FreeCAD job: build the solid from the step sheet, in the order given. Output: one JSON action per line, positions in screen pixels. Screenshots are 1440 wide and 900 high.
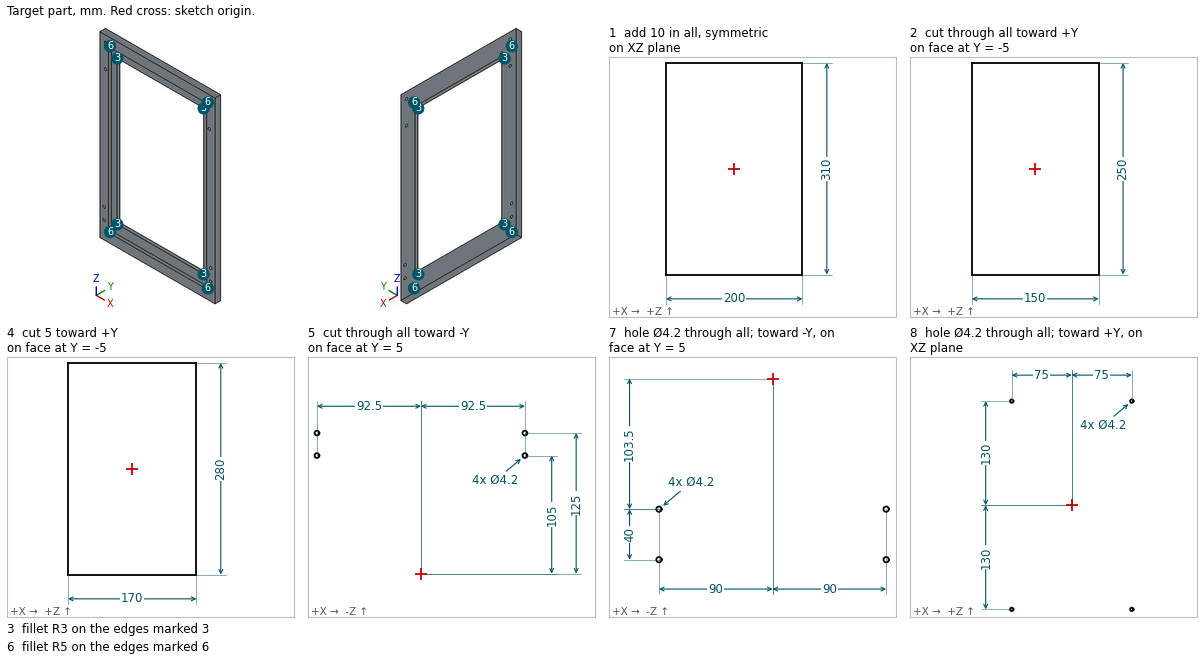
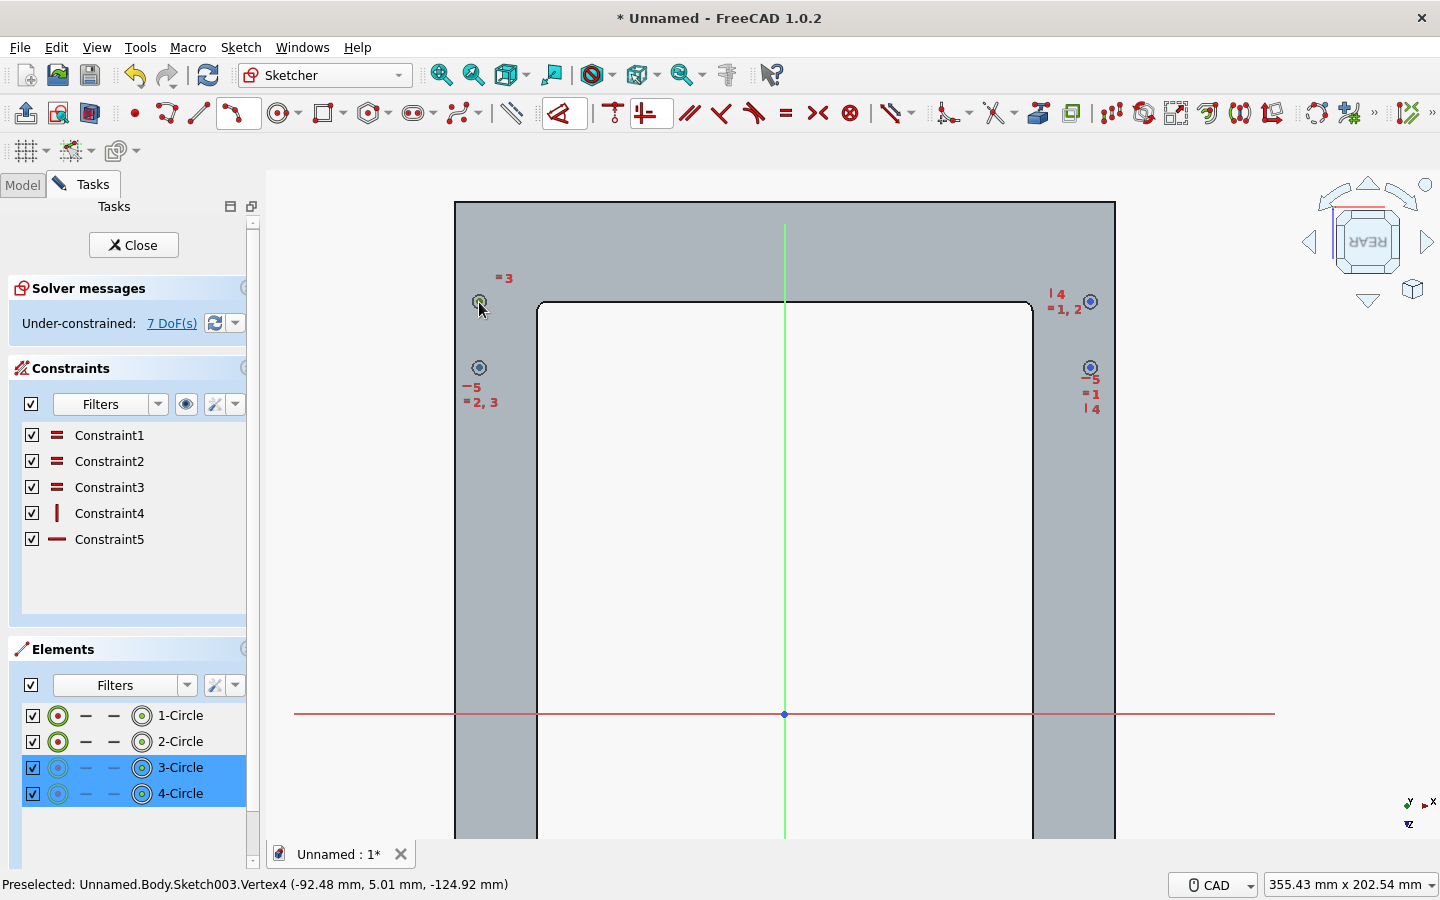
{"action": "key", "text": "v"}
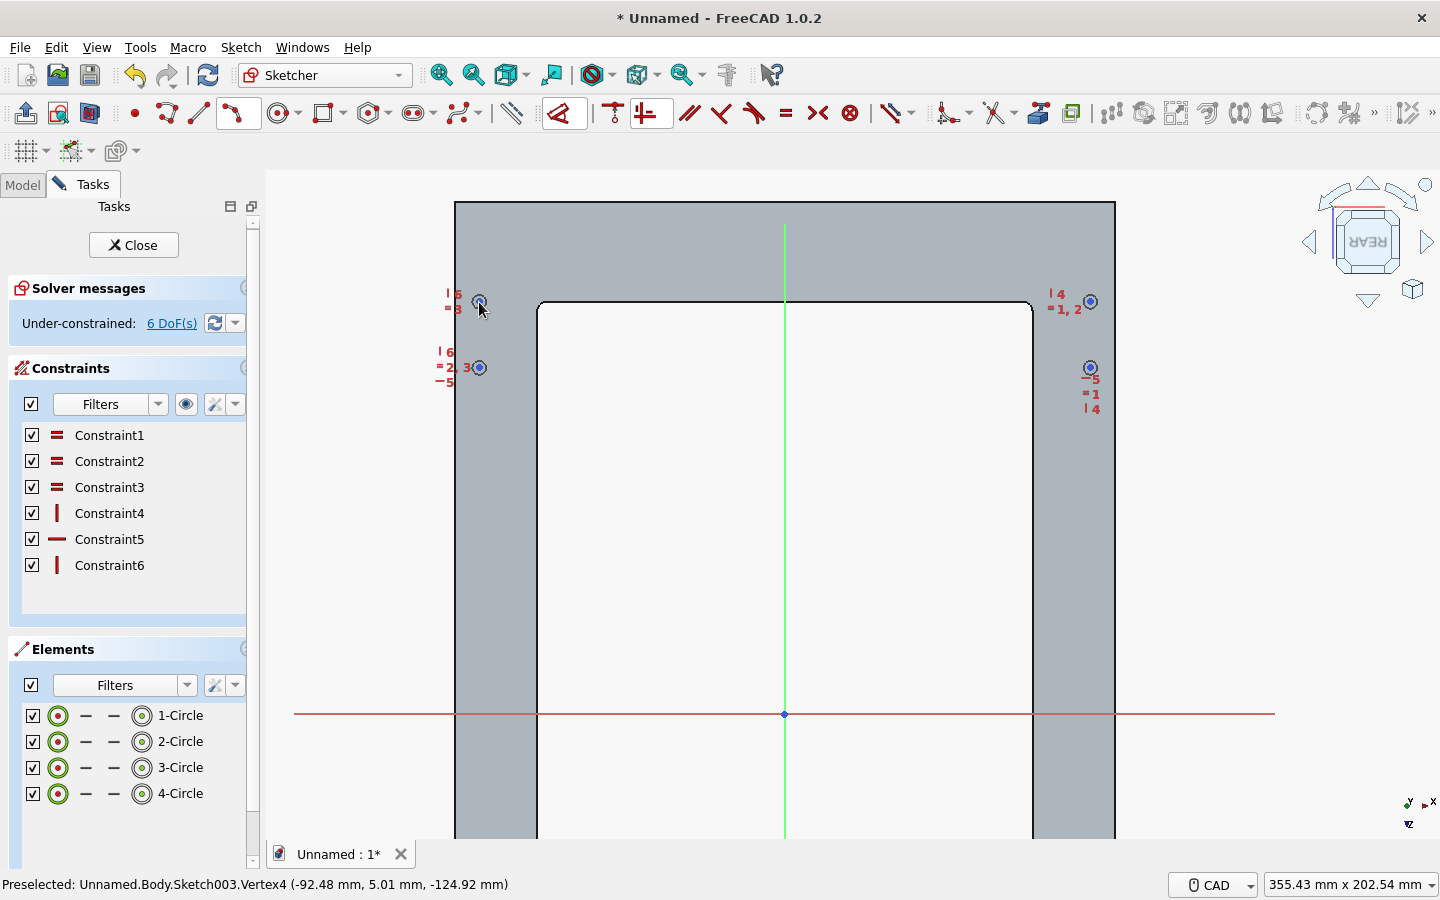
{"action": "left_click", "coordinate": [1090, 302]}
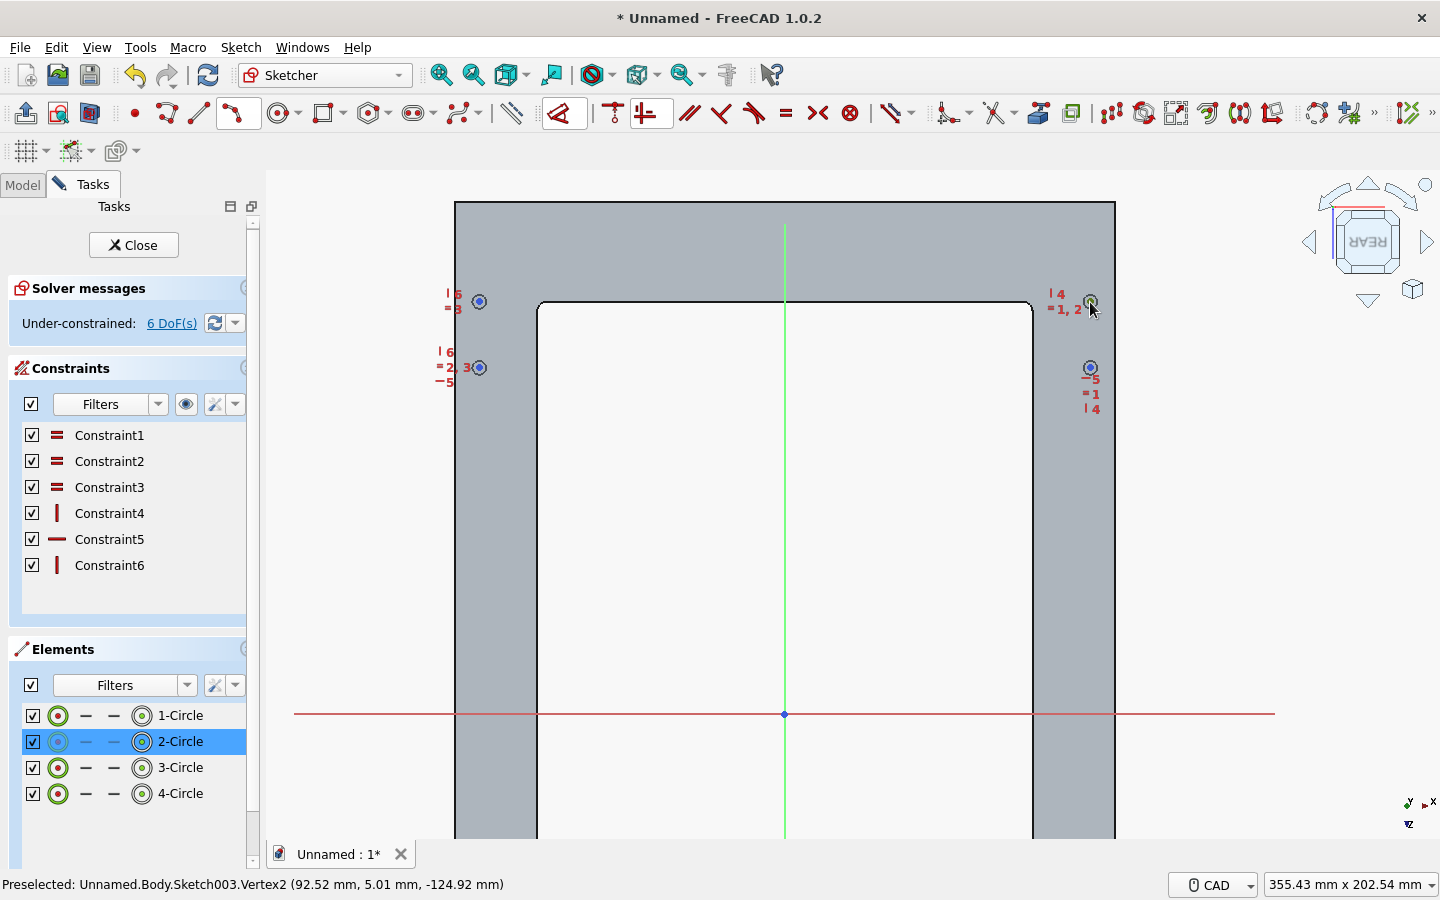
{"action": "left_click", "coordinate": [479, 302]}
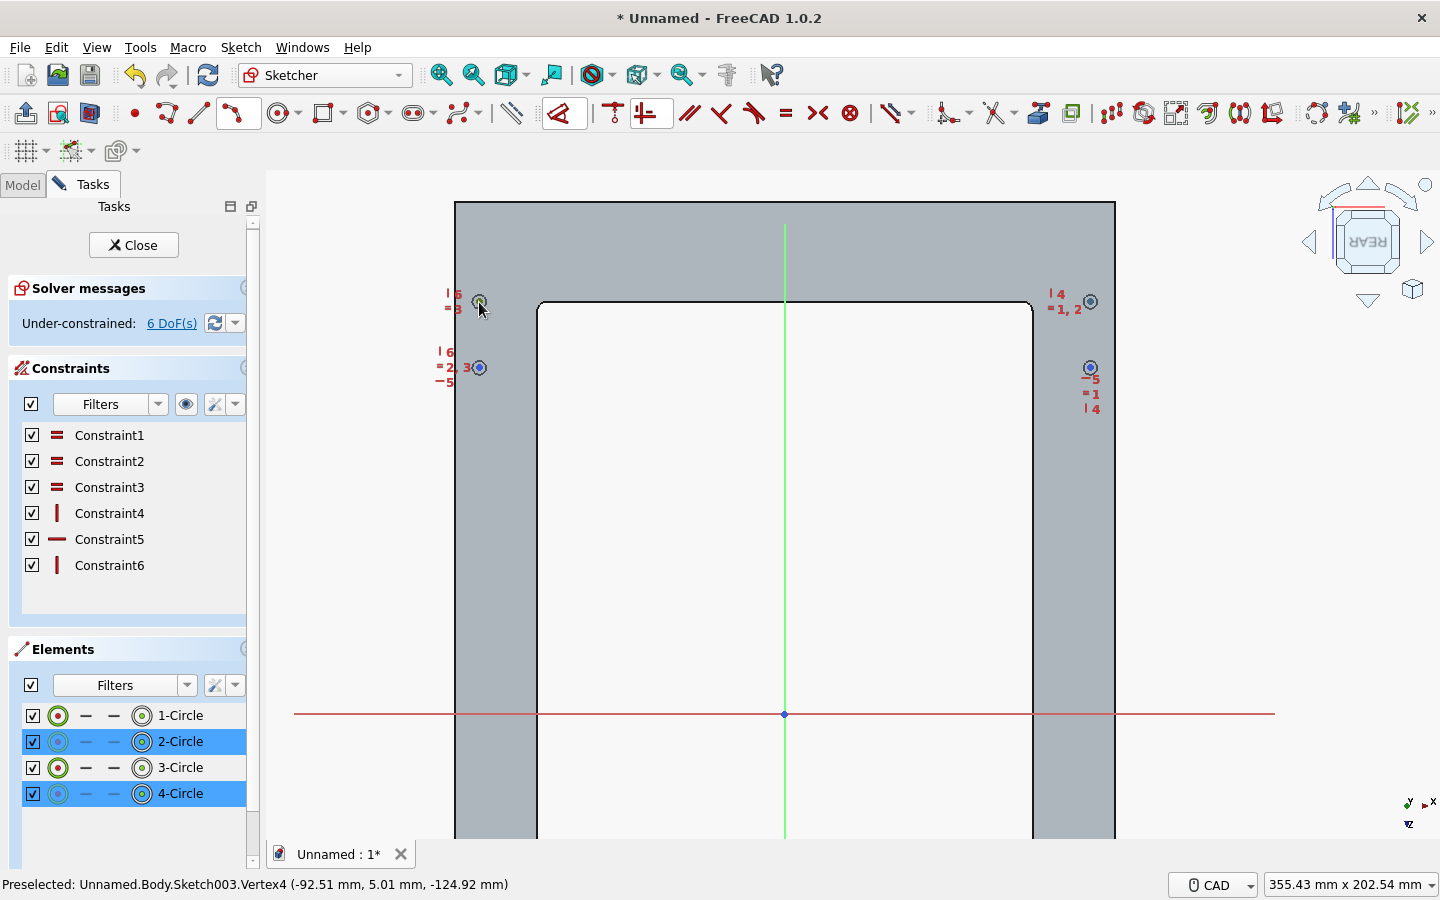
{"action": "key", "text": "h"}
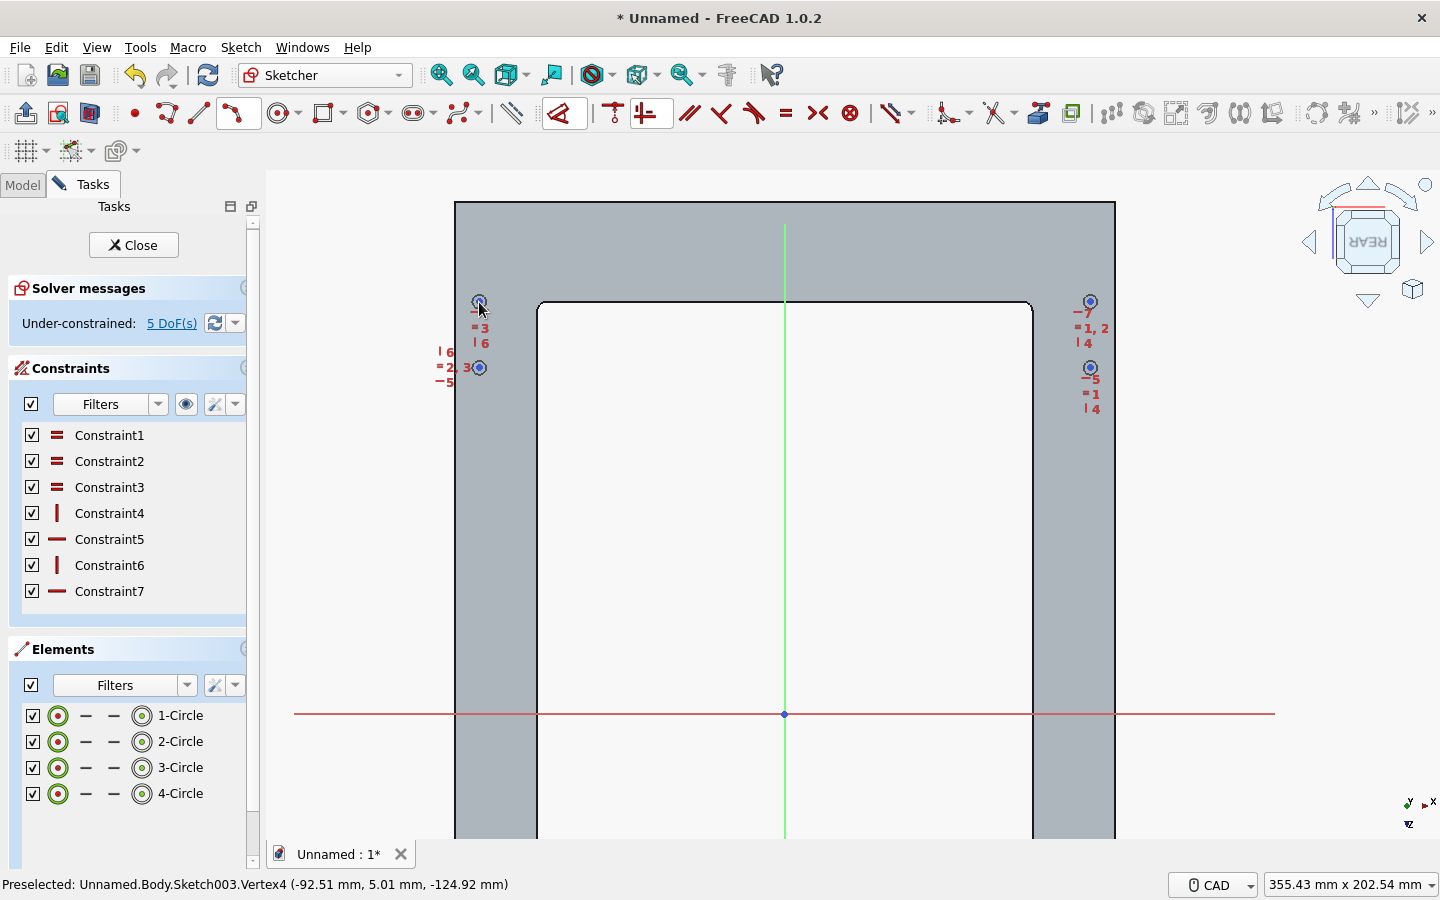
{"action": "scroll", "coordinate": [1091, 361], "scroll_direction": "up", "scroll_amount": 6}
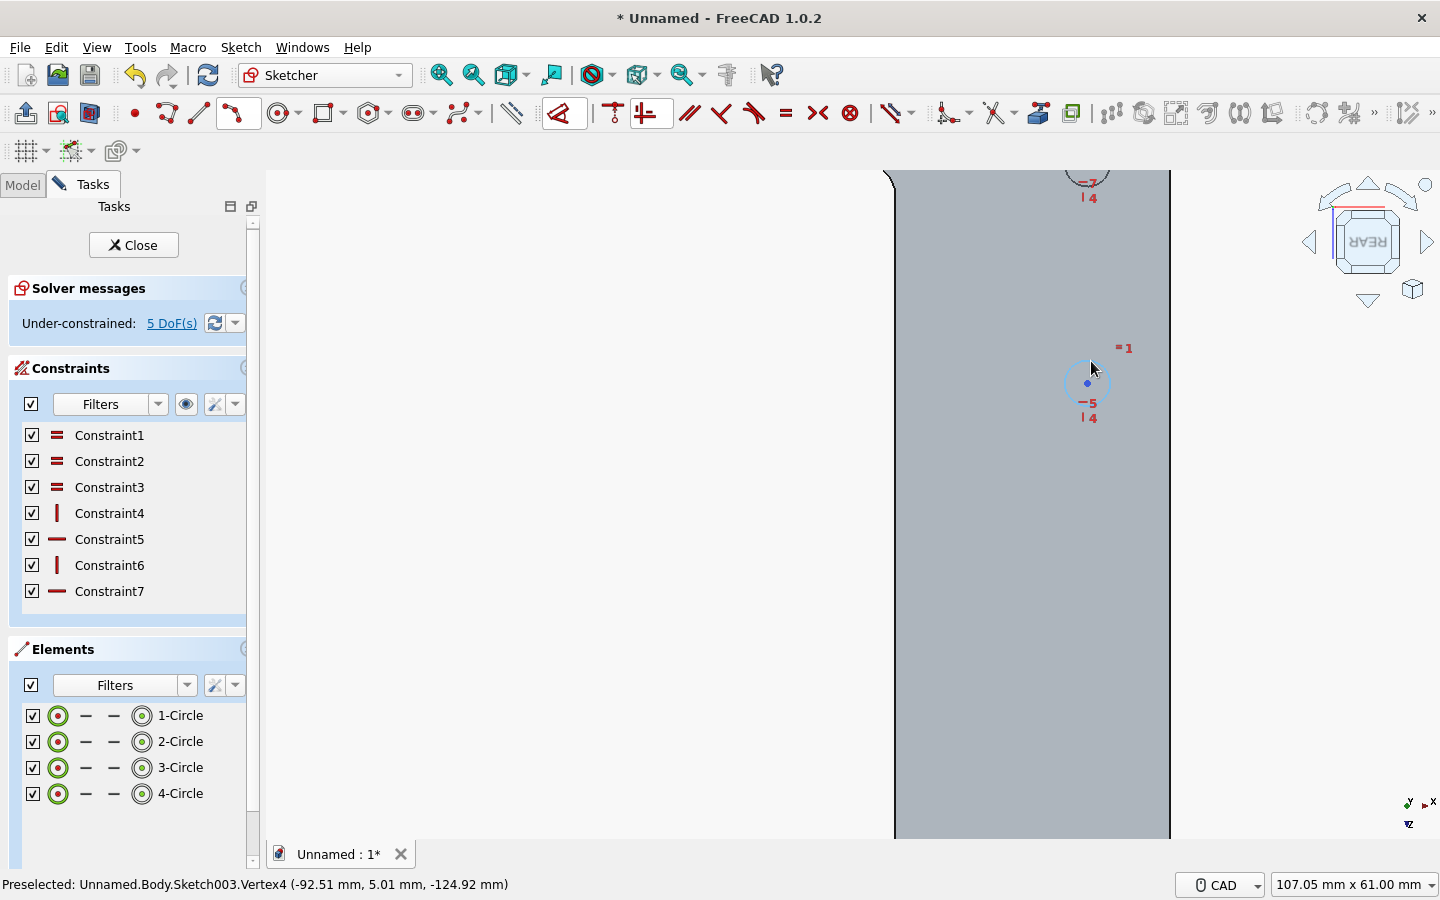
{"action": "left_click", "coordinate": [1088, 361]}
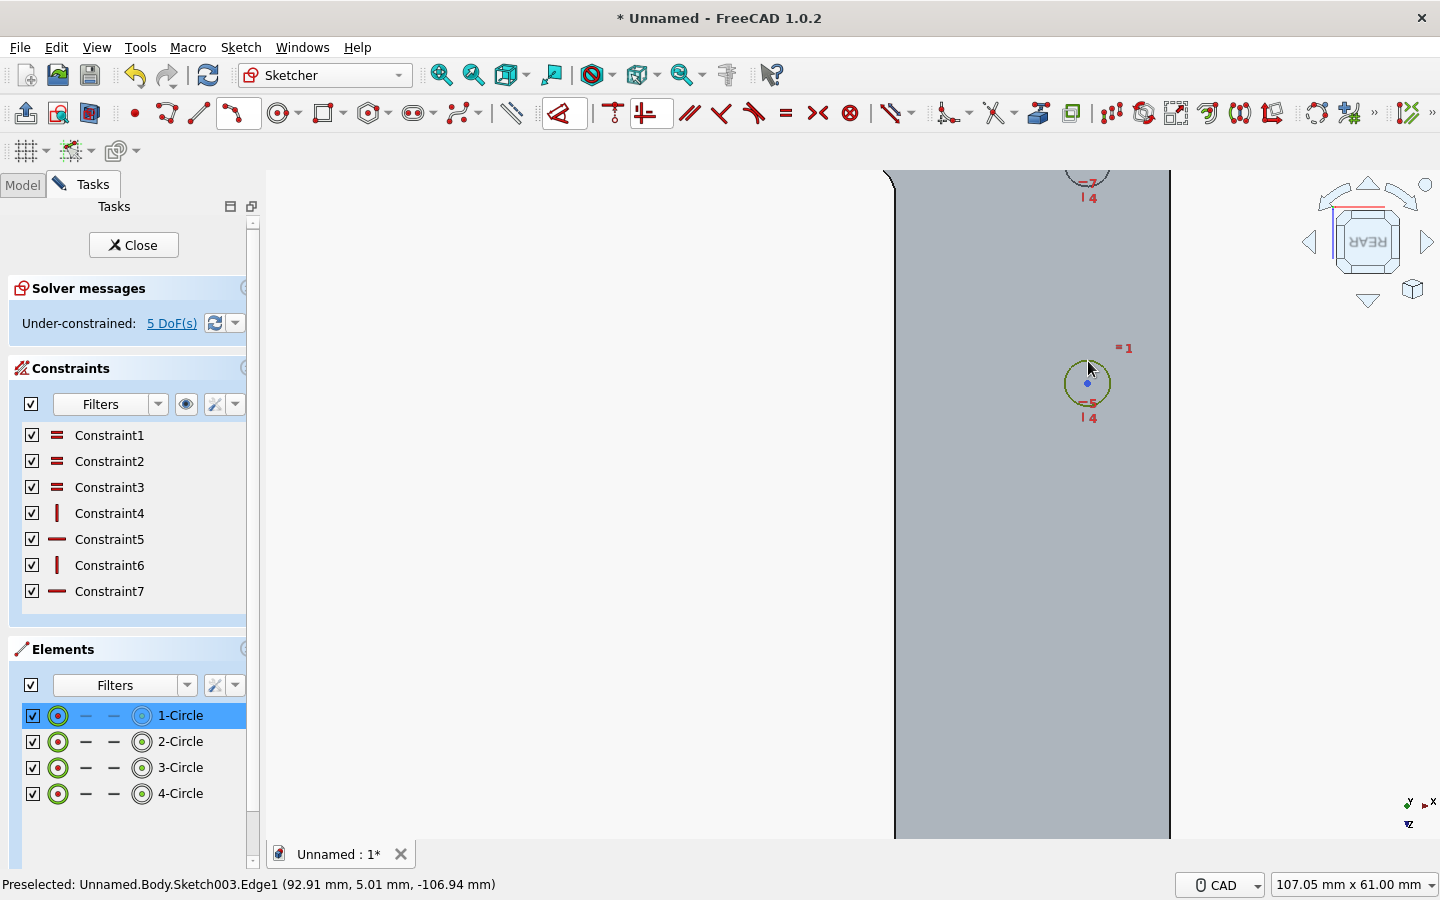
{"action": "key", "text": "k o"}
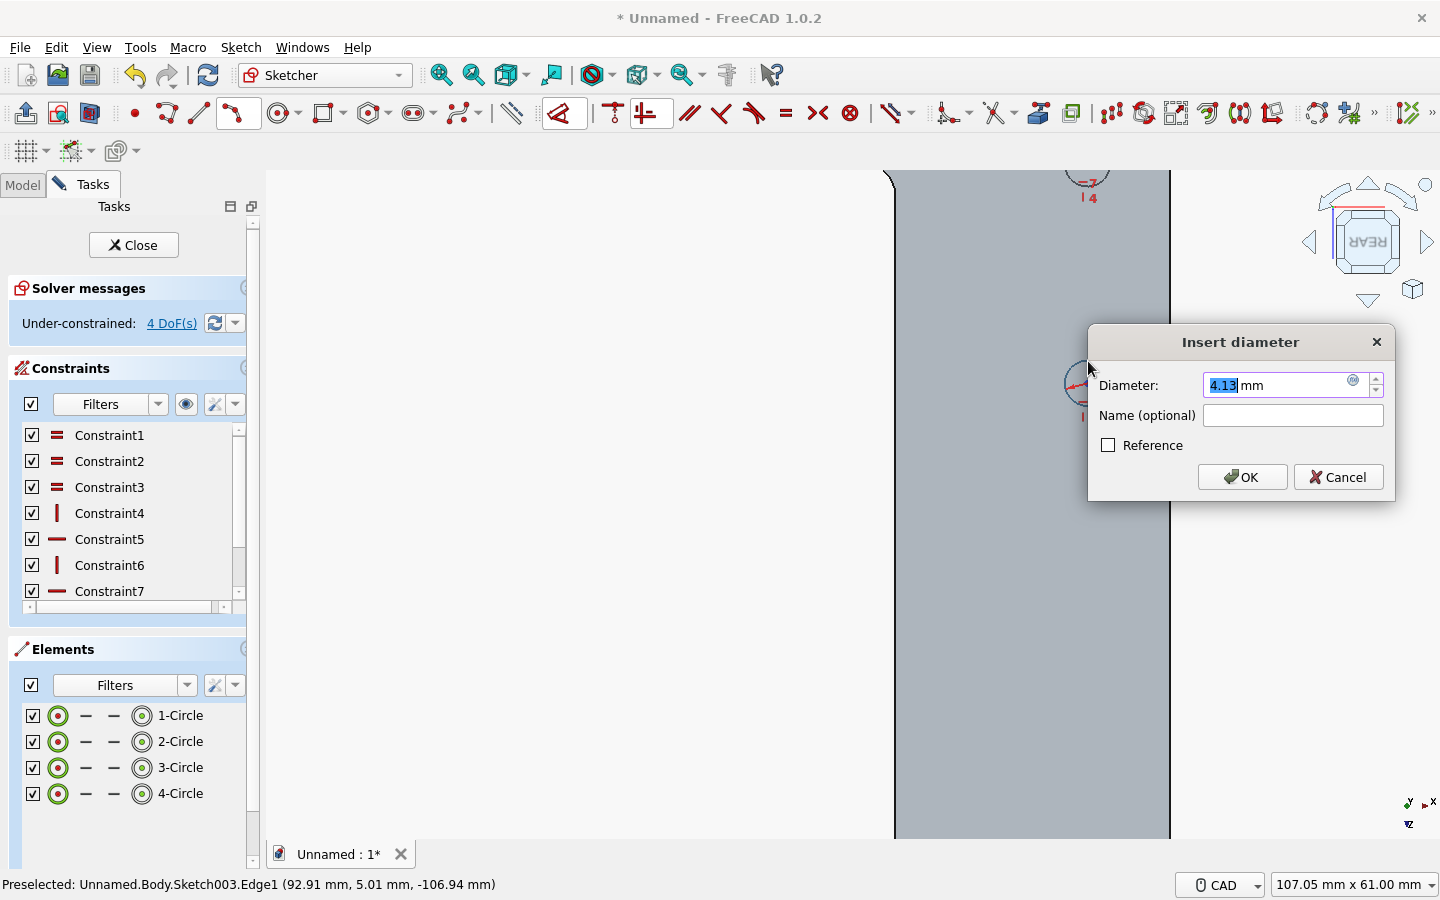
{"action": "type", "text": "4.2"}
{"action": "key", "text": "Return"}